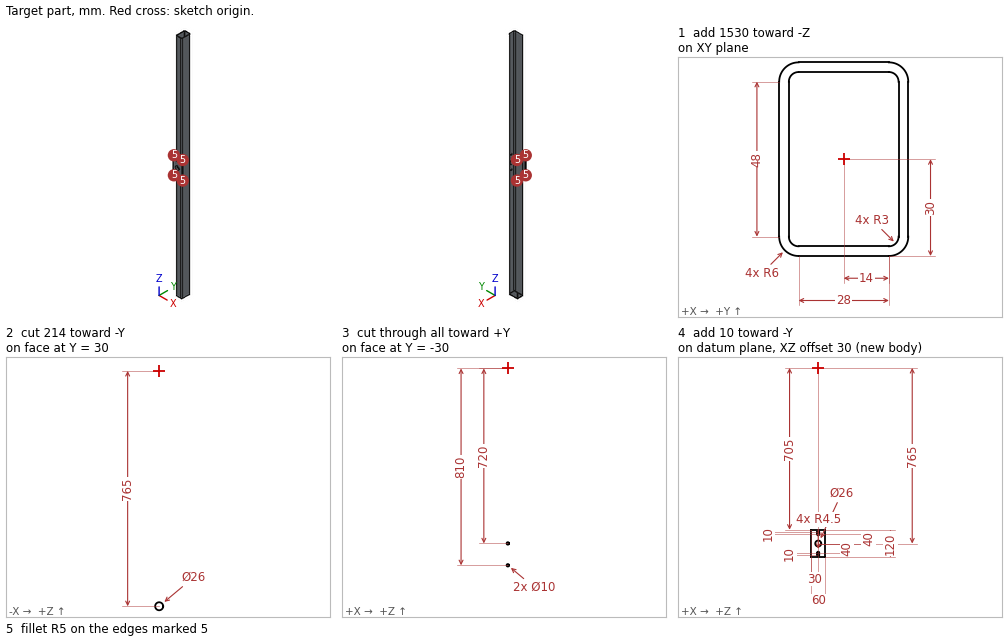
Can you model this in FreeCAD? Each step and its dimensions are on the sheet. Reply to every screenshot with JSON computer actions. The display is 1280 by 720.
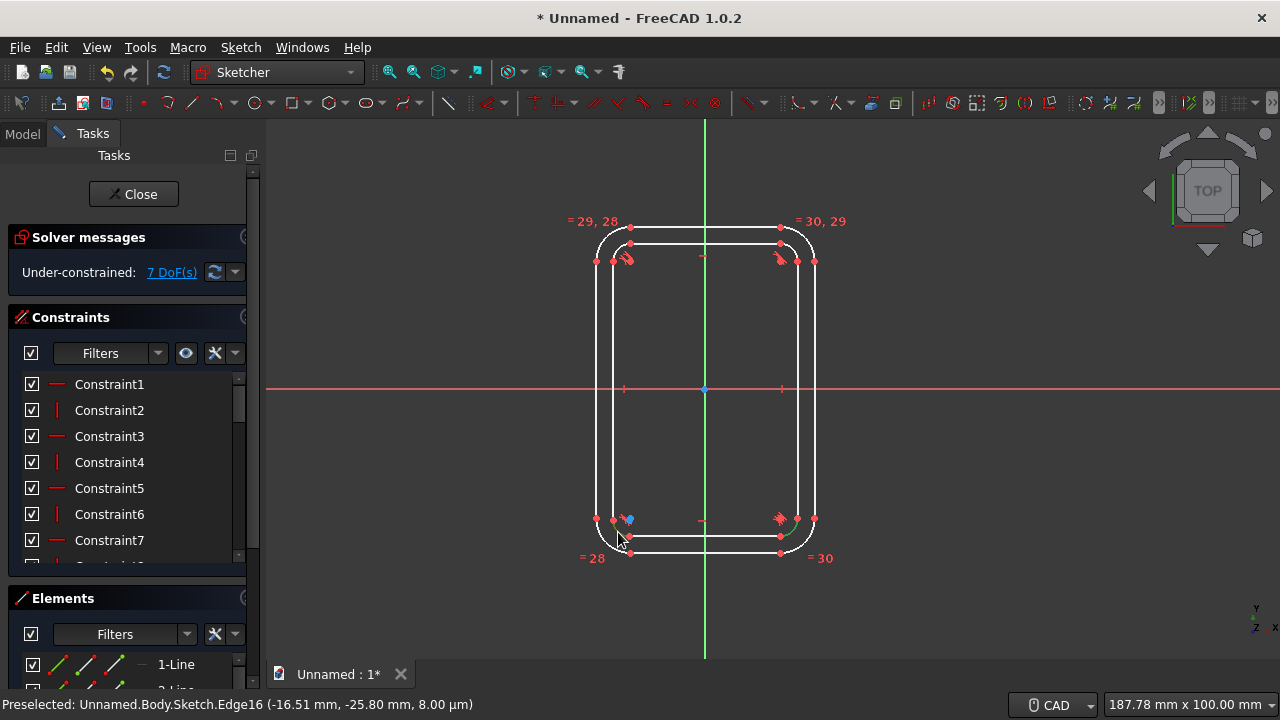
{"action": "left_click", "coordinate": [668, 104]}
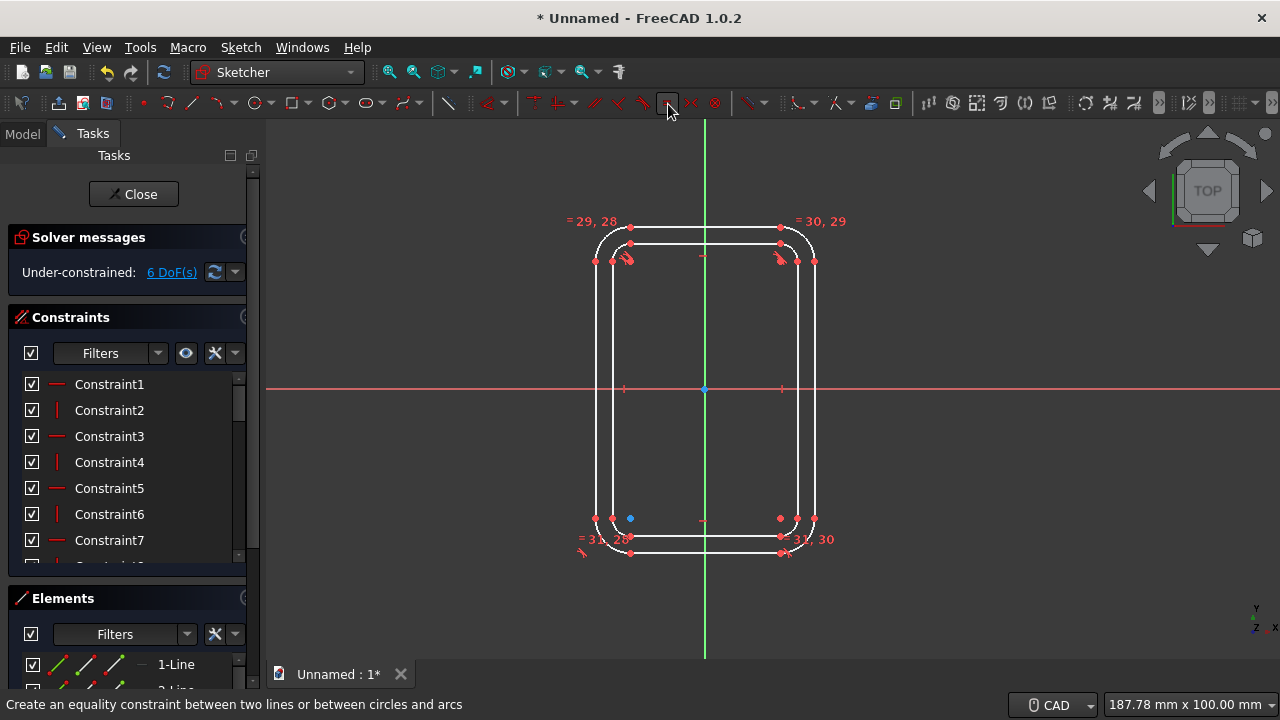
{"action": "left_click", "coordinate": [488, 104]}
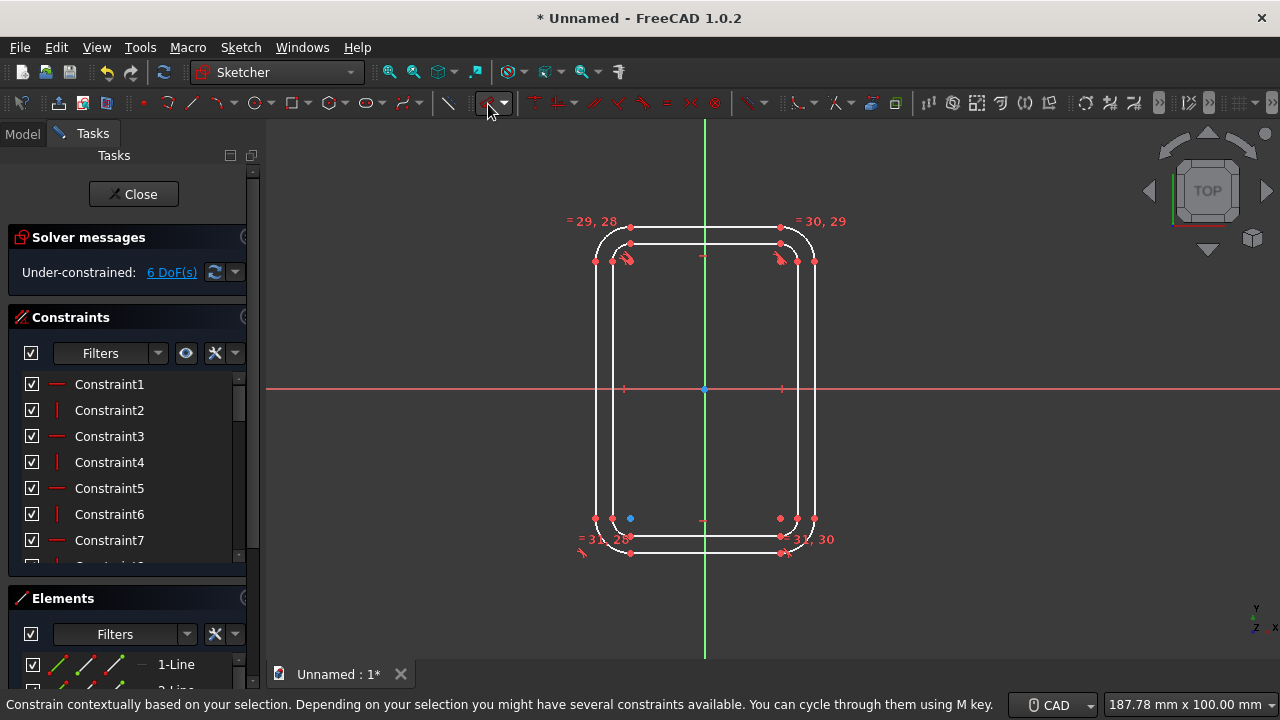
{"action": "scroll", "coordinate": [599, 534], "scroll_direction": "up", "scroll_amount": 2}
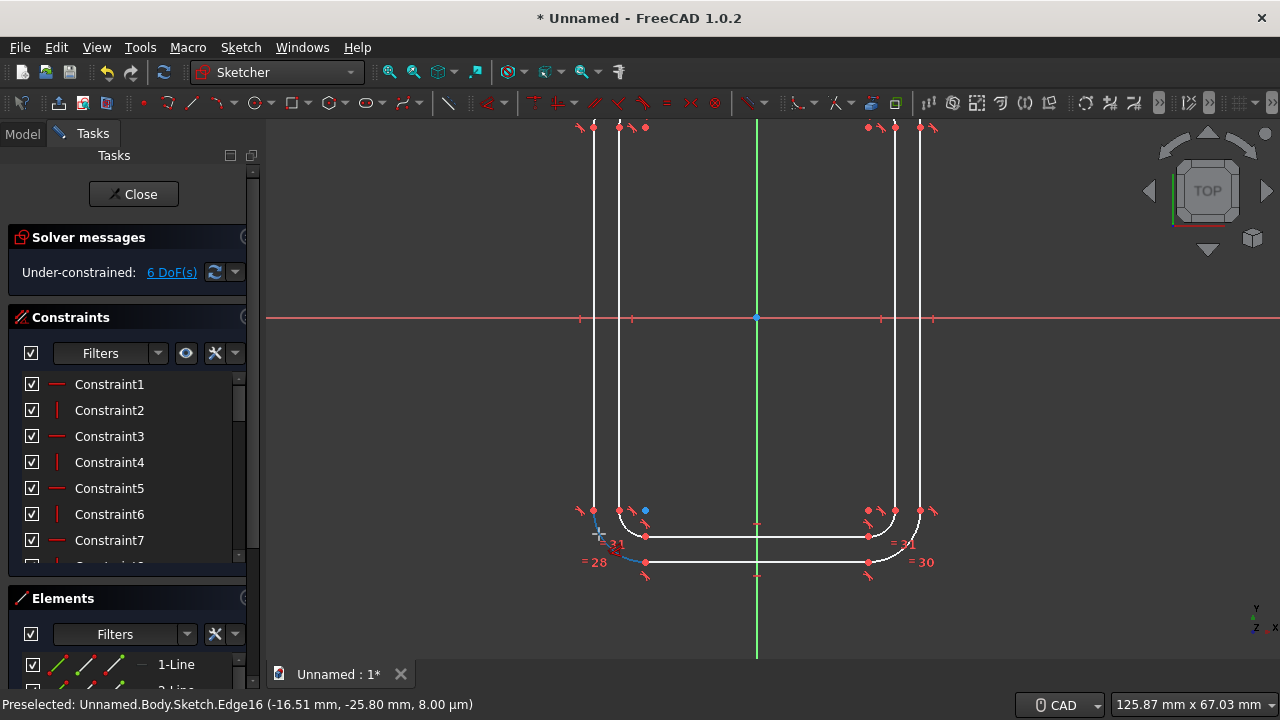
{"action": "left_click", "coordinate": [600, 534]}
{"action": "left_click", "coordinate": [572, 549]}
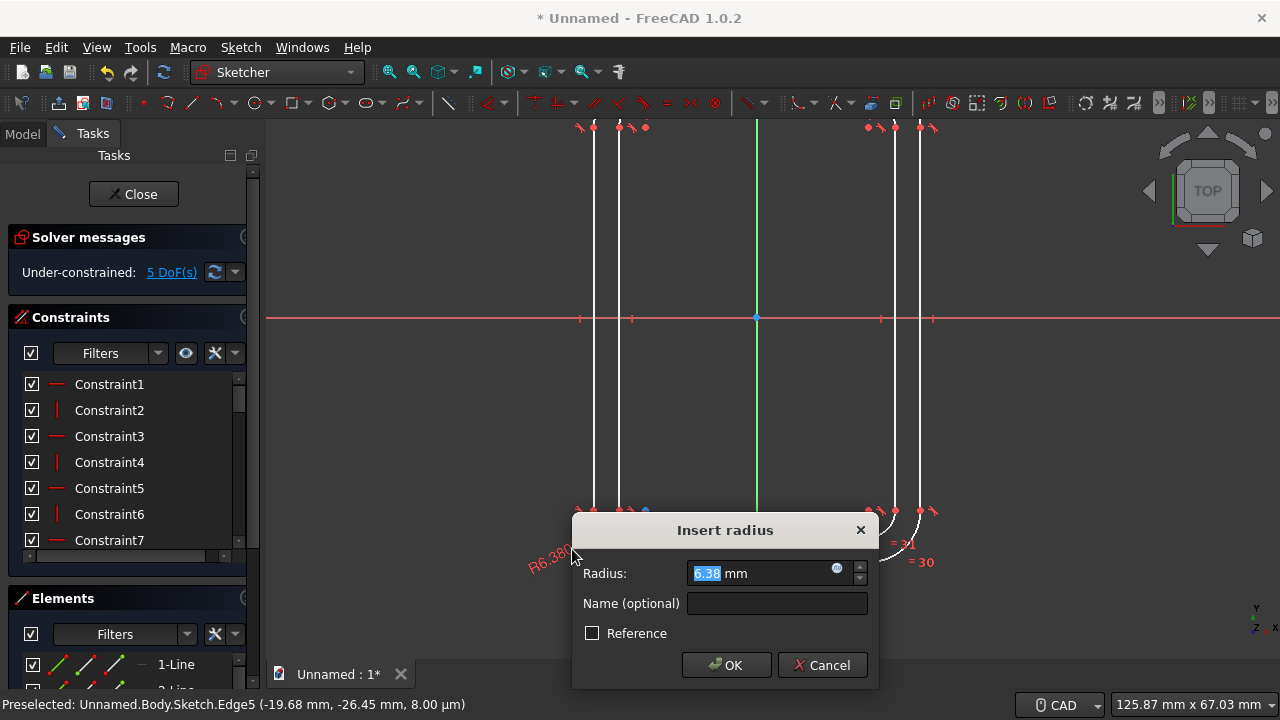
{"action": "type", "text": "6"}
{"action": "key", "text": "Return"}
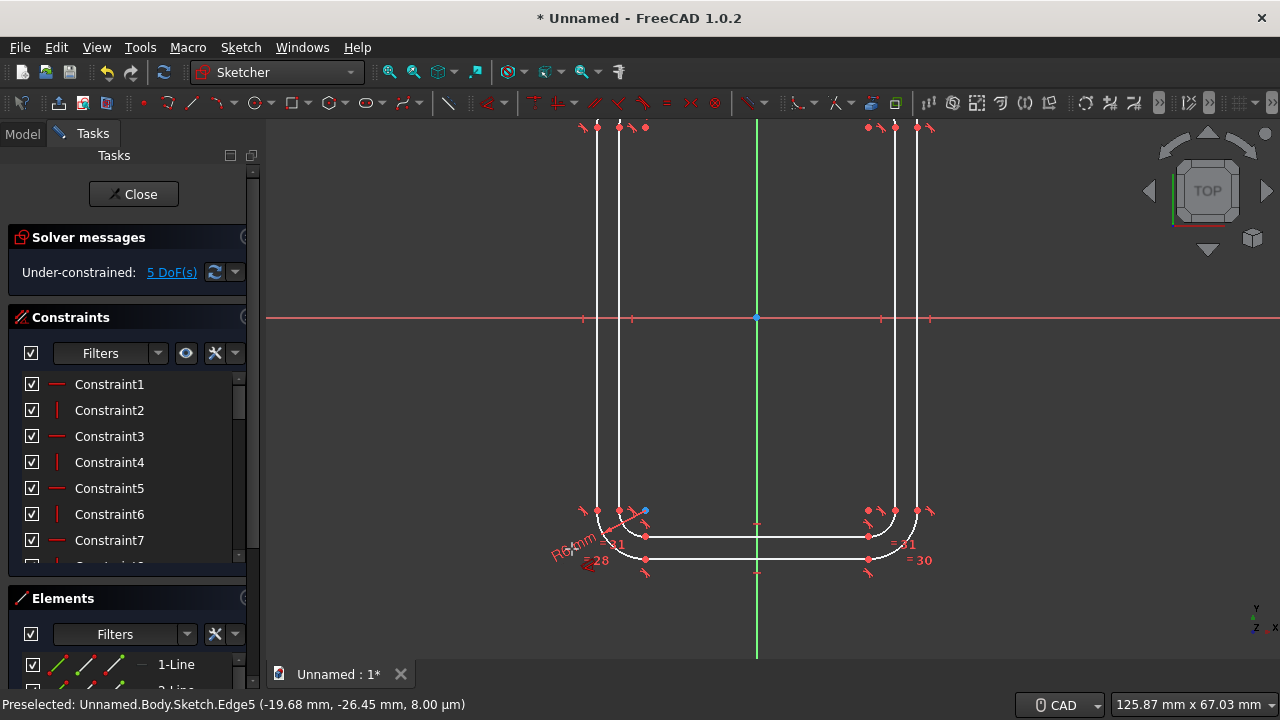
{"action": "scroll", "coordinate": [881, 534], "scroll_direction": "up", "scroll_amount": 3}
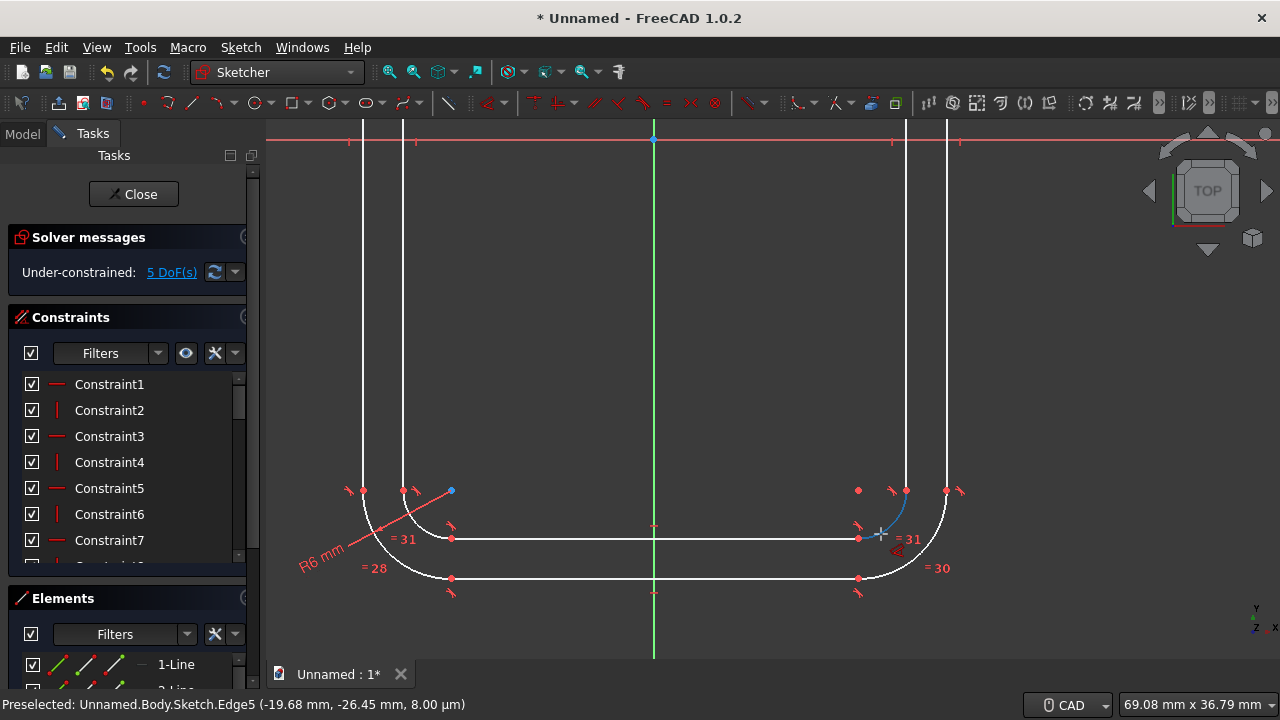
{"action": "left_click", "coordinate": [880, 533]}
{"action": "left_click", "coordinate": [819, 559]}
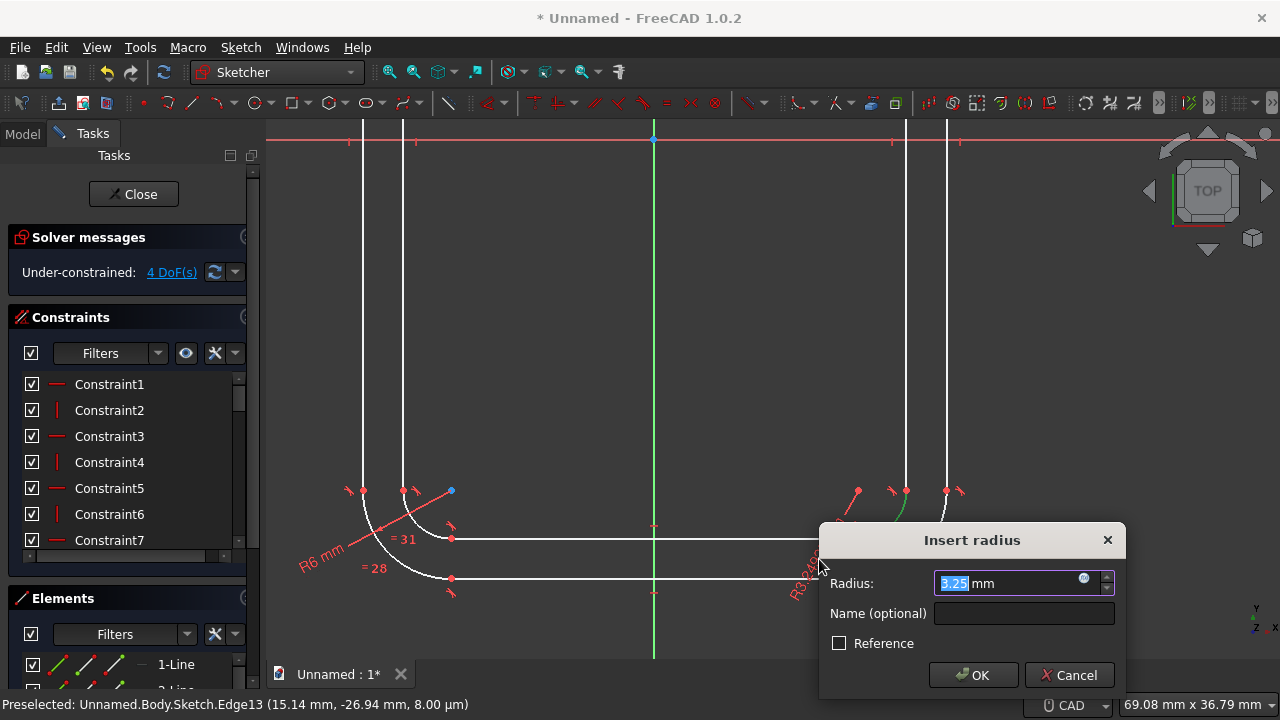
{"action": "type", "text": "3"}
{"action": "key", "text": "Return"}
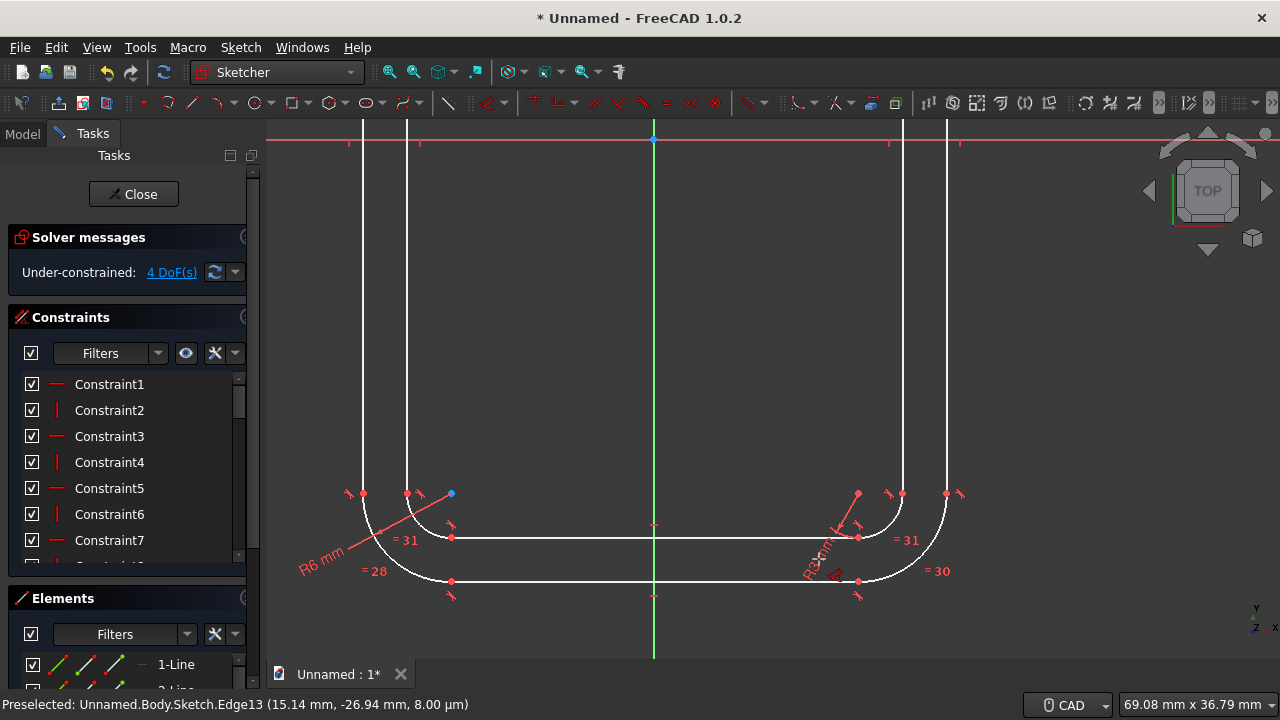
{"action": "left_click", "coordinate": [736, 582]}
{"action": "left_click", "coordinate": [561, 616]}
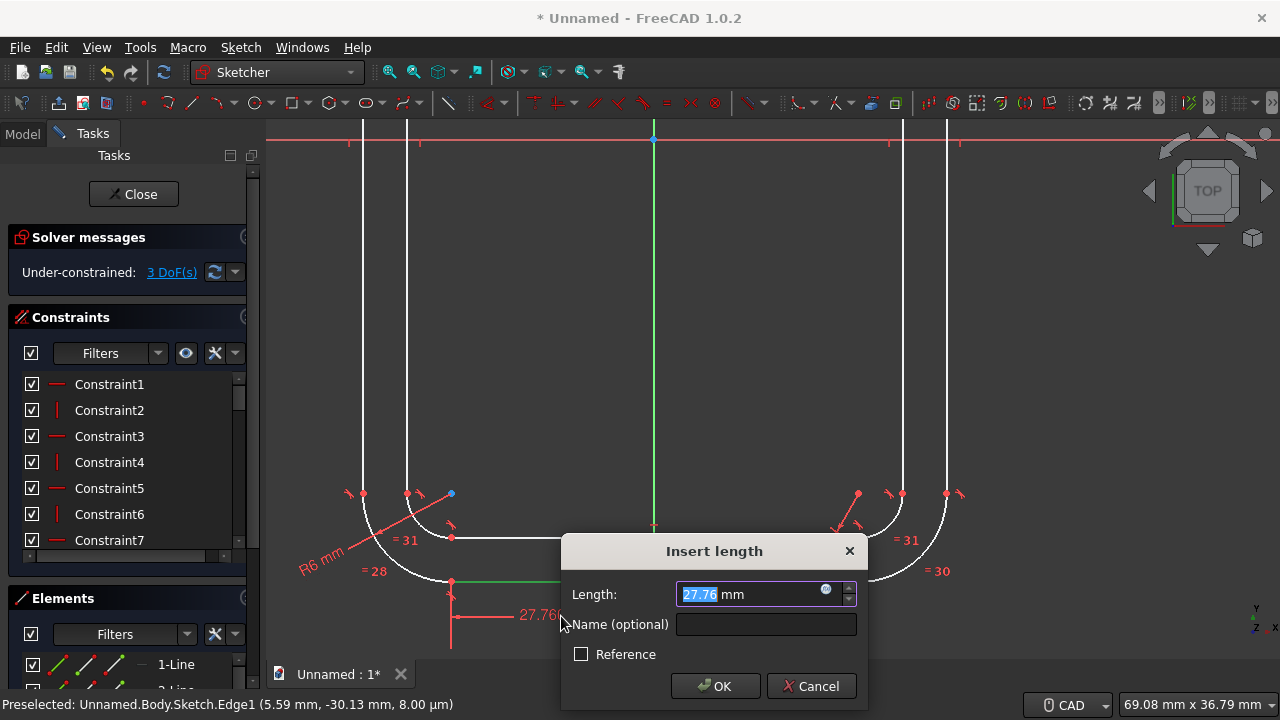
{"action": "type", "text": "28"}
{"action": "key", "text": "Return"}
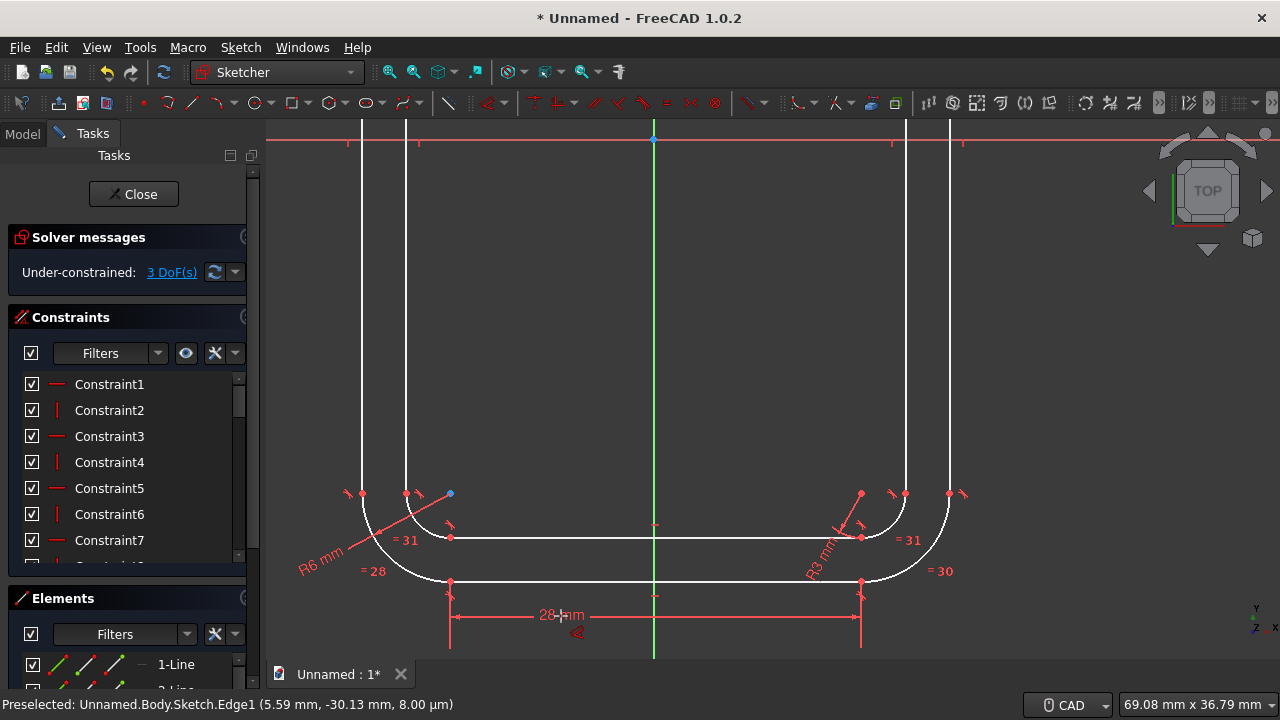
{"action": "left_click", "coordinate": [362, 283]}
{"action": "left_click", "coordinate": [328, 320]}